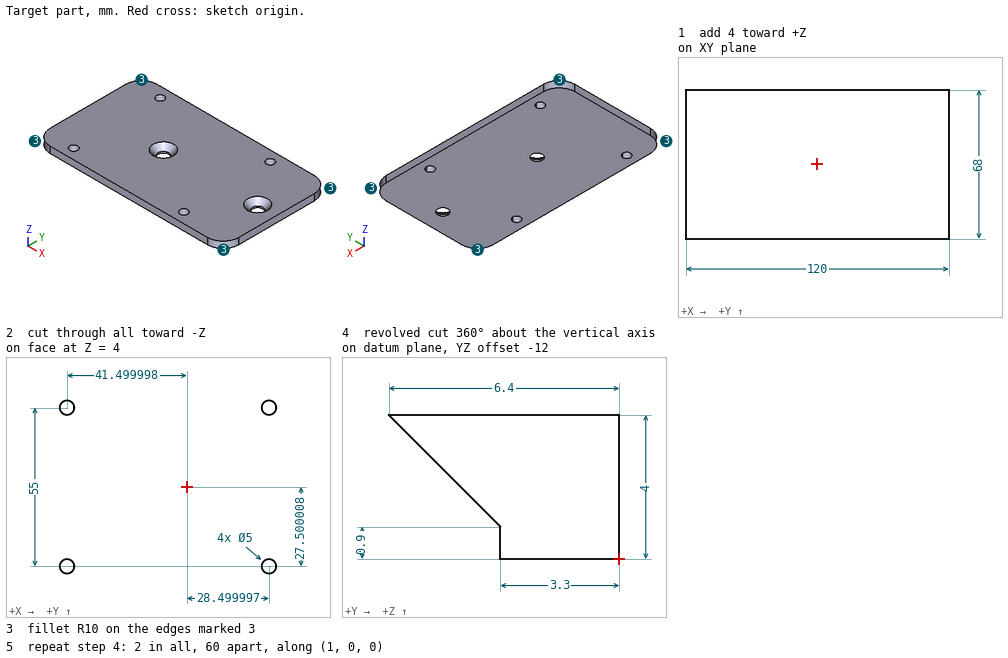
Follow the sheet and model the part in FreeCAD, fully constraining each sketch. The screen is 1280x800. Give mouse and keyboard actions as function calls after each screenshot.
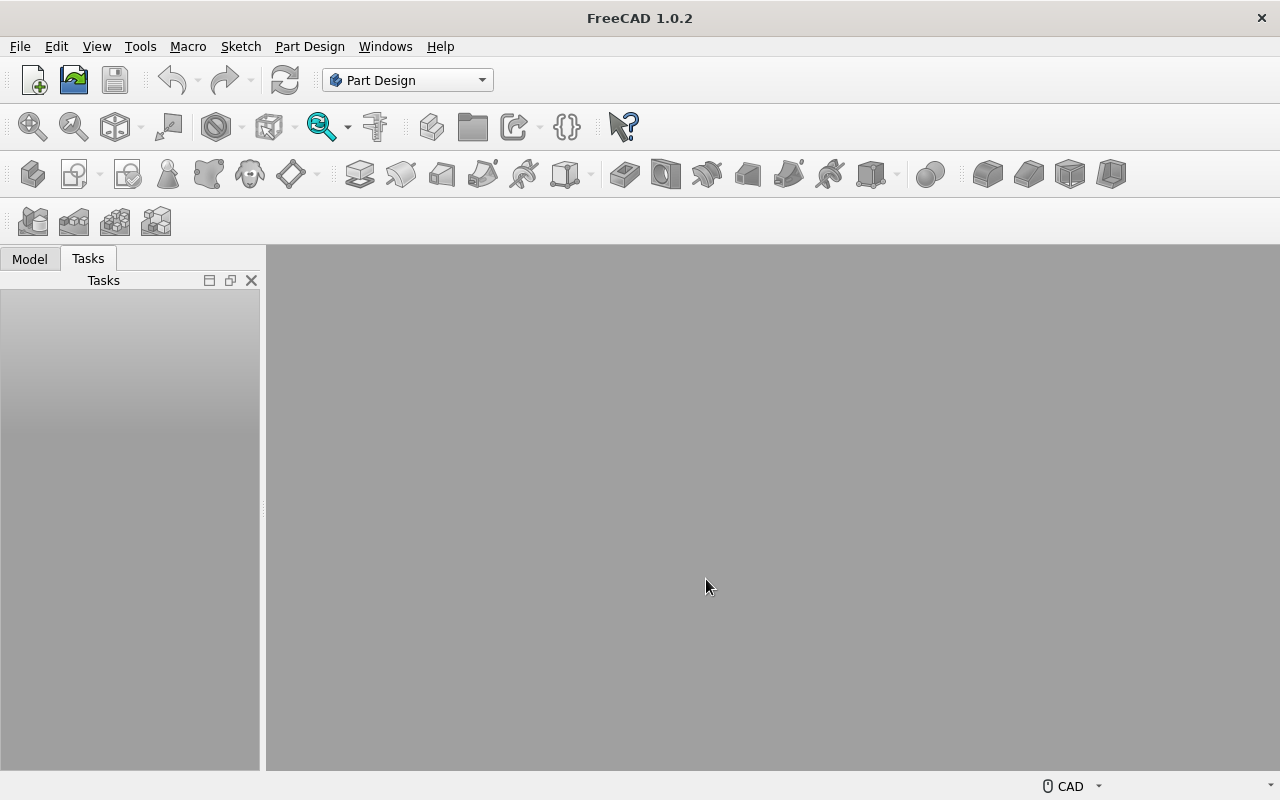
click(33, 80)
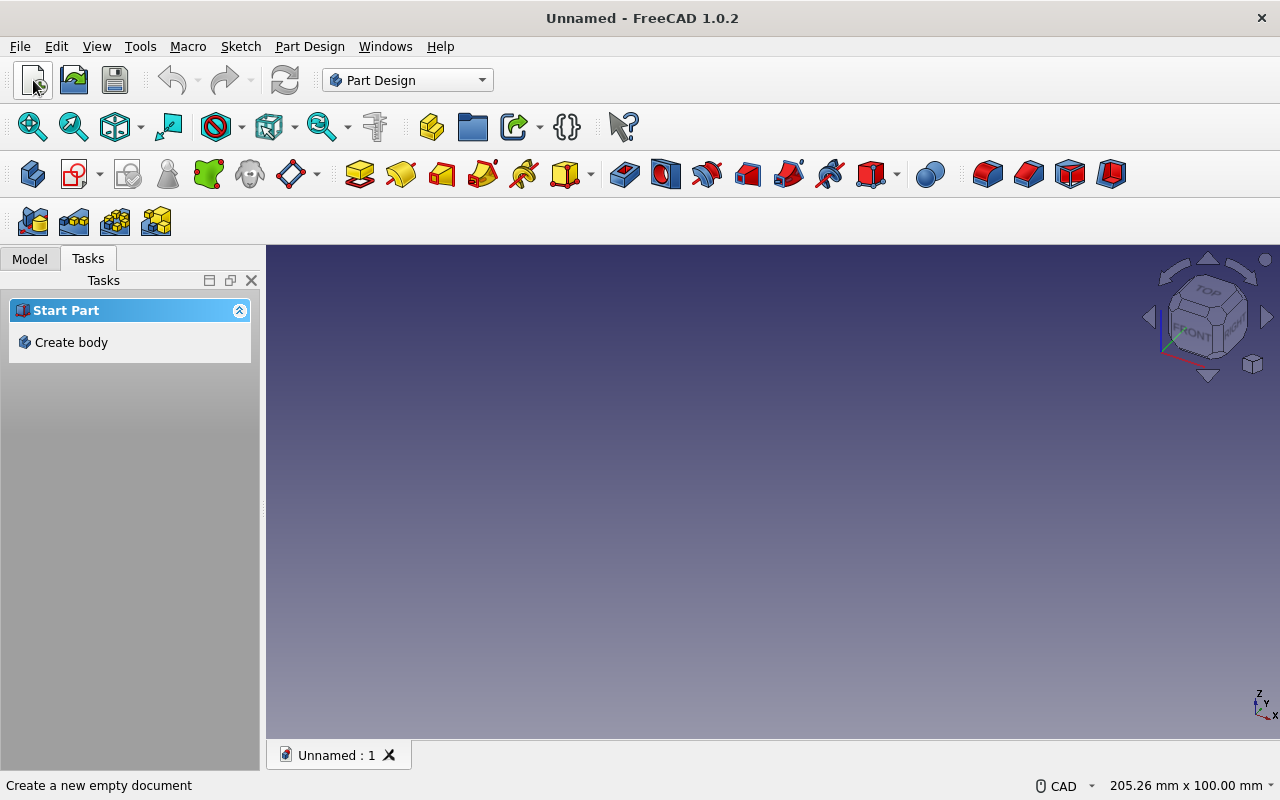
click(74, 174)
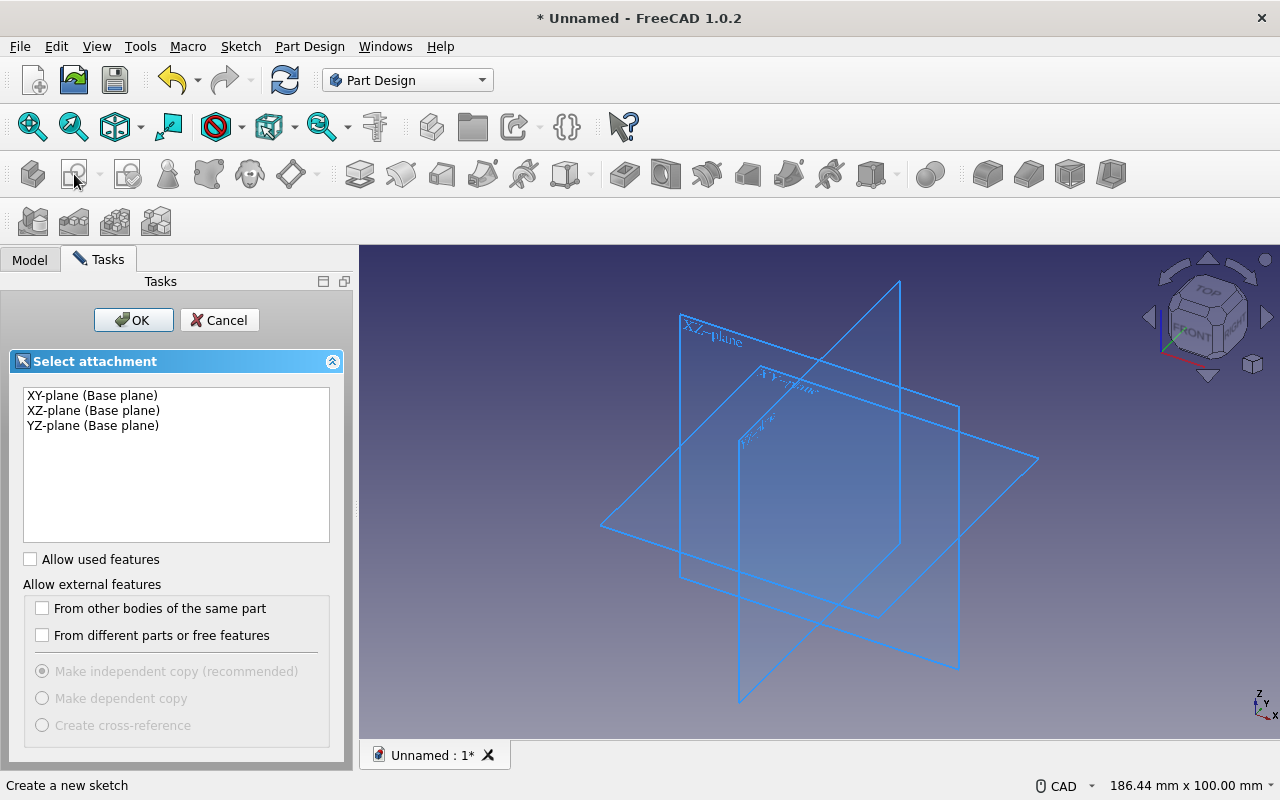
click(84, 396)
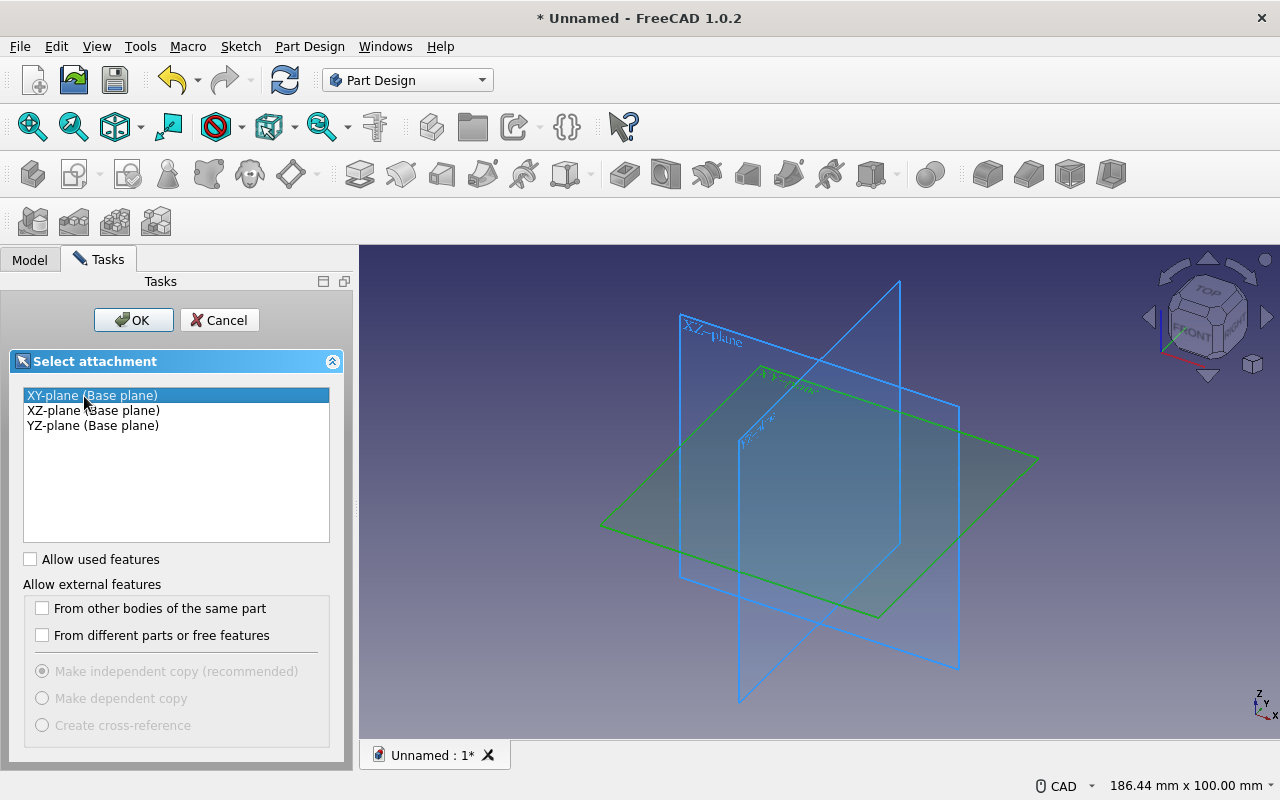
click(134, 320)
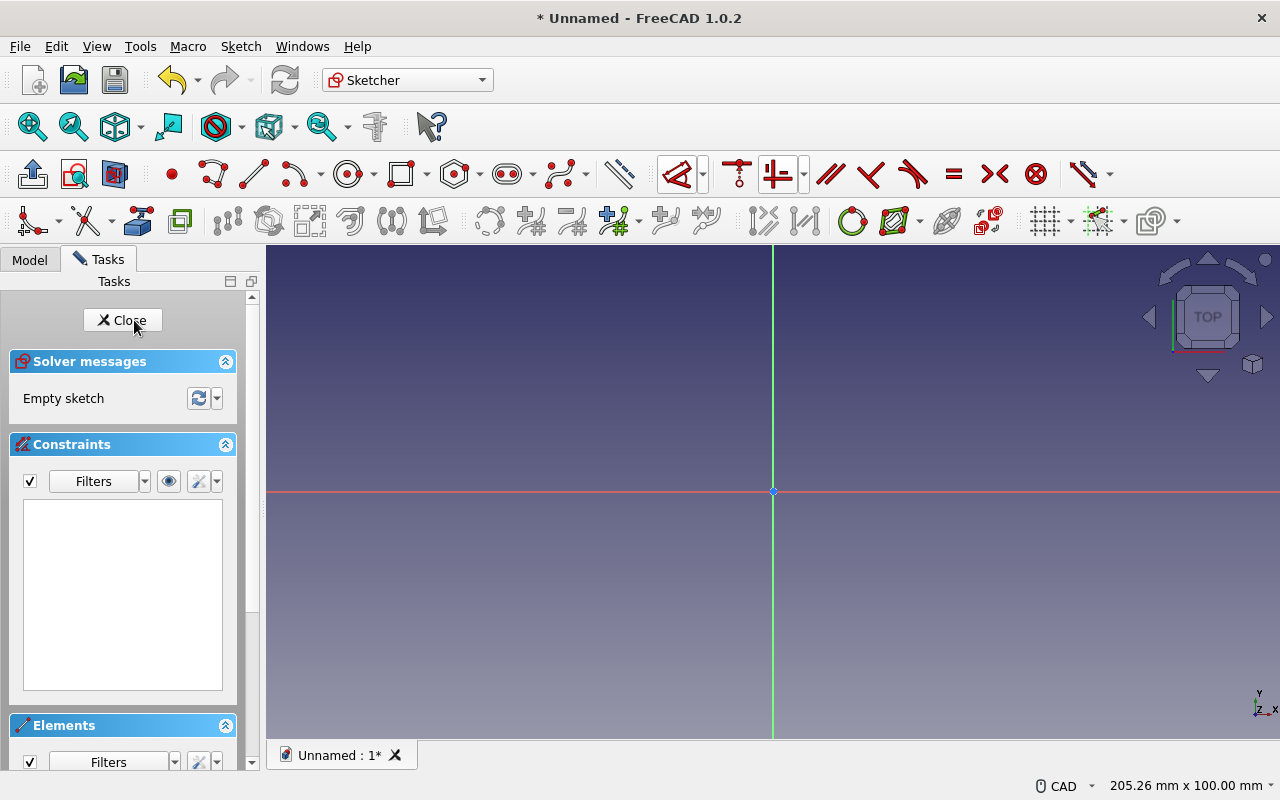
click(426, 174)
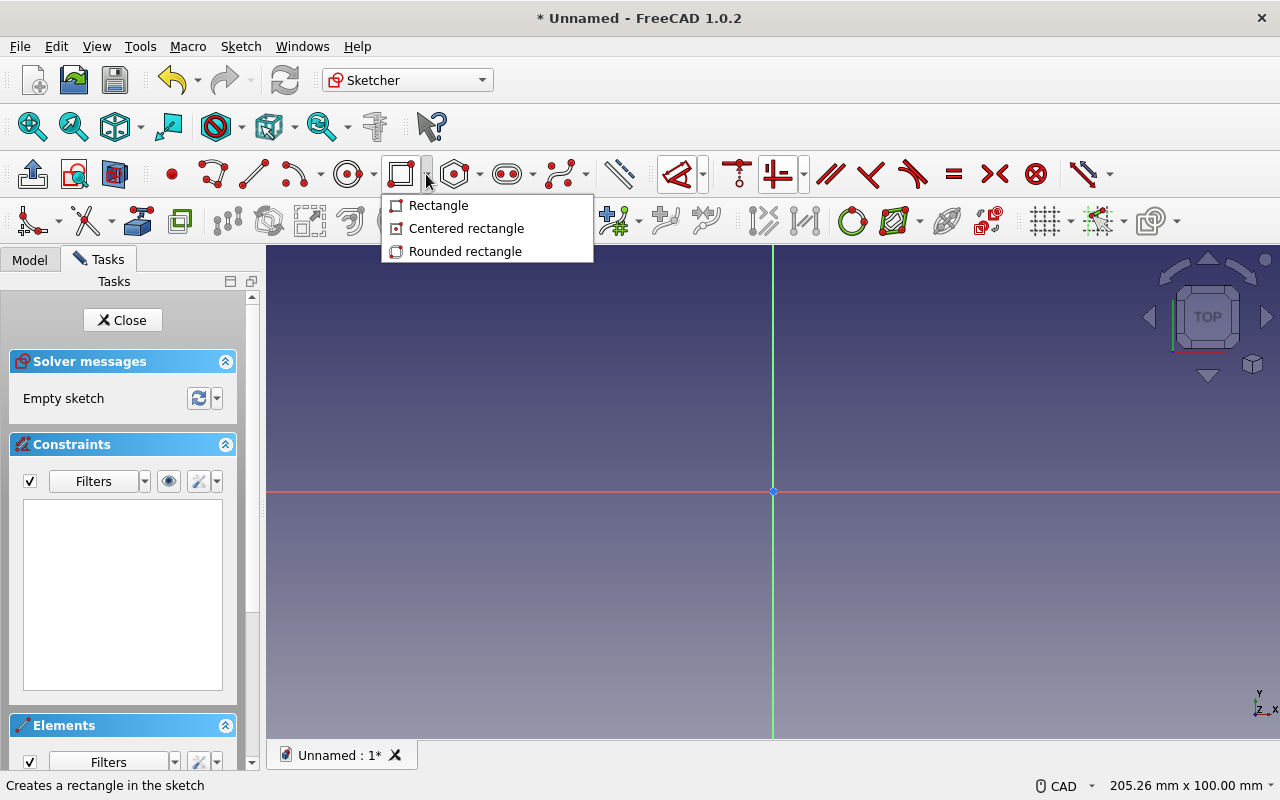
click(488, 228)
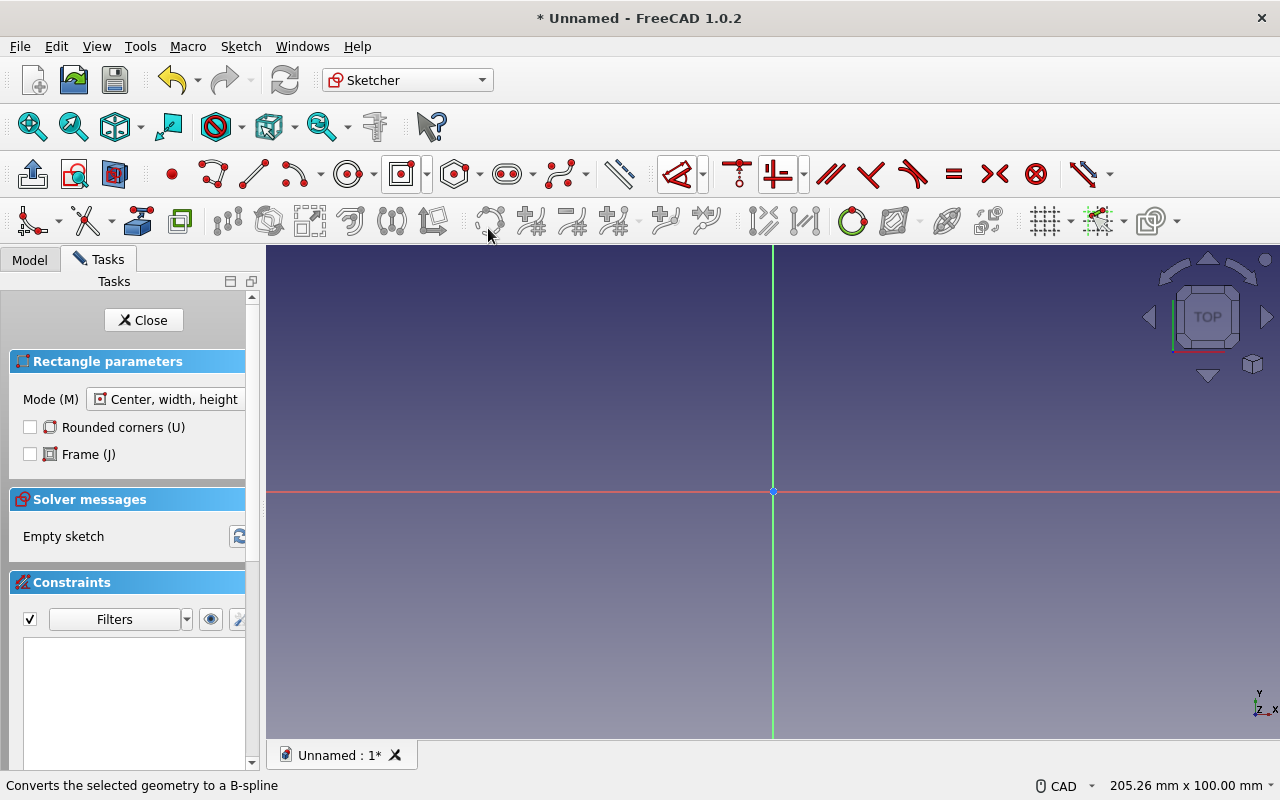
click(773, 492)
move(1069, 324)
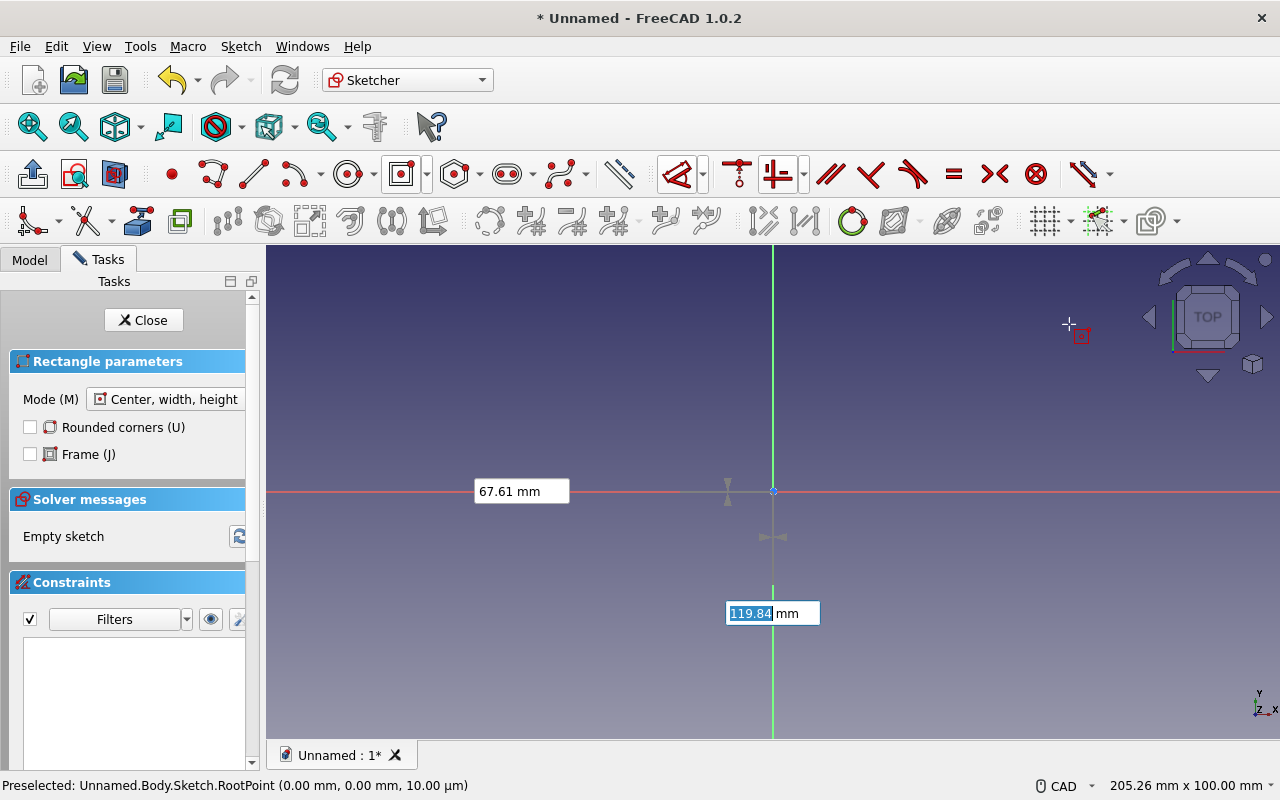
text(120)
key(Tab)
text(68)
key(Return)
key(Escape)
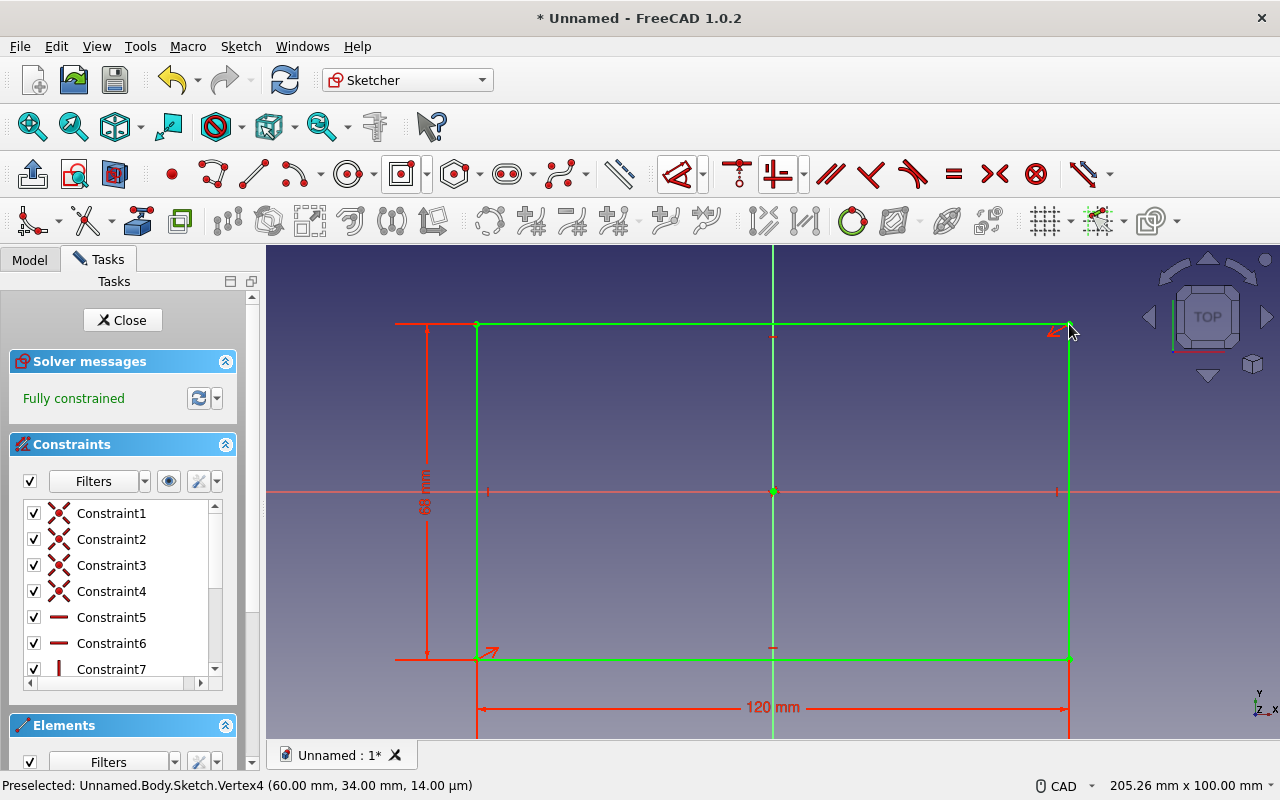
click(123, 320)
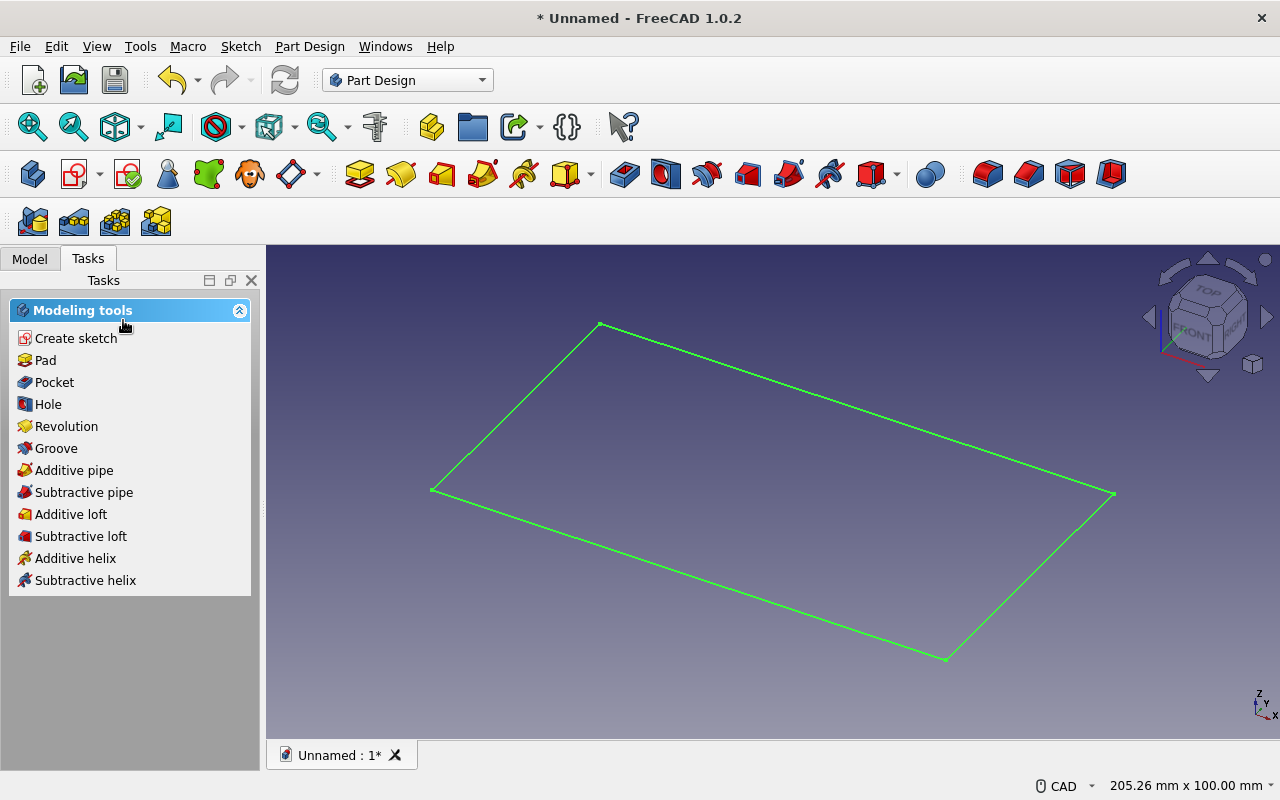
click(360, 174)